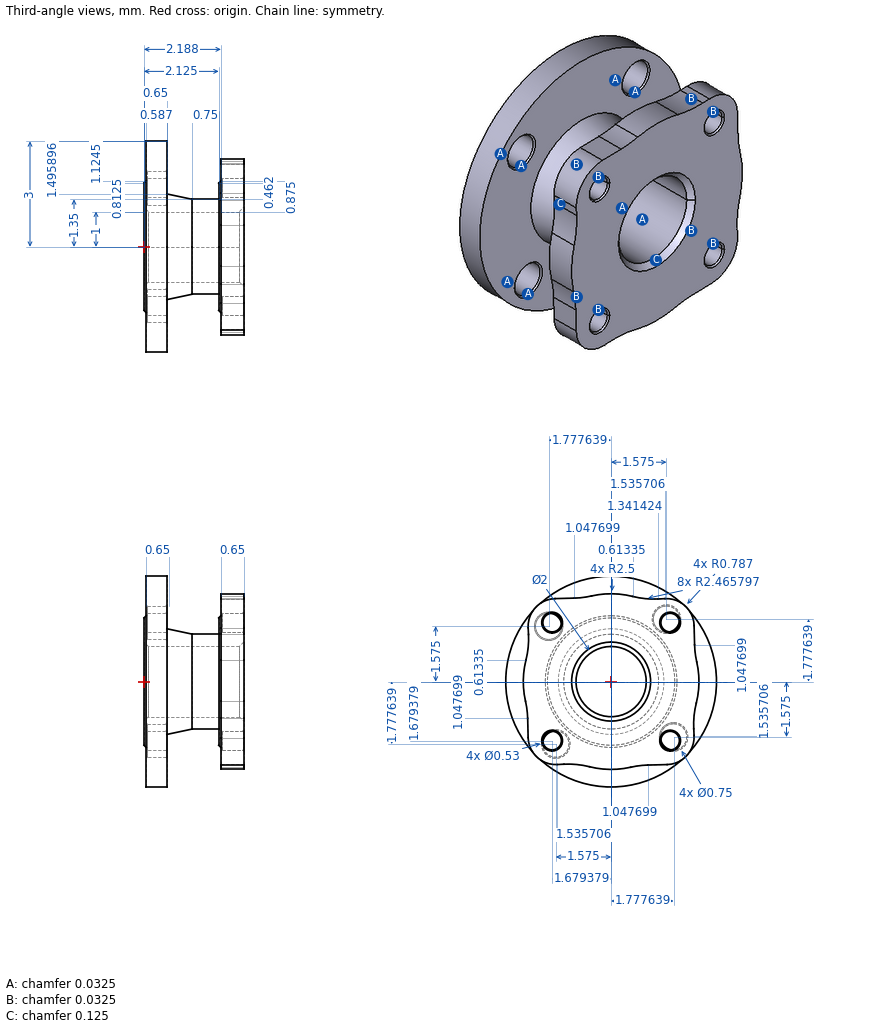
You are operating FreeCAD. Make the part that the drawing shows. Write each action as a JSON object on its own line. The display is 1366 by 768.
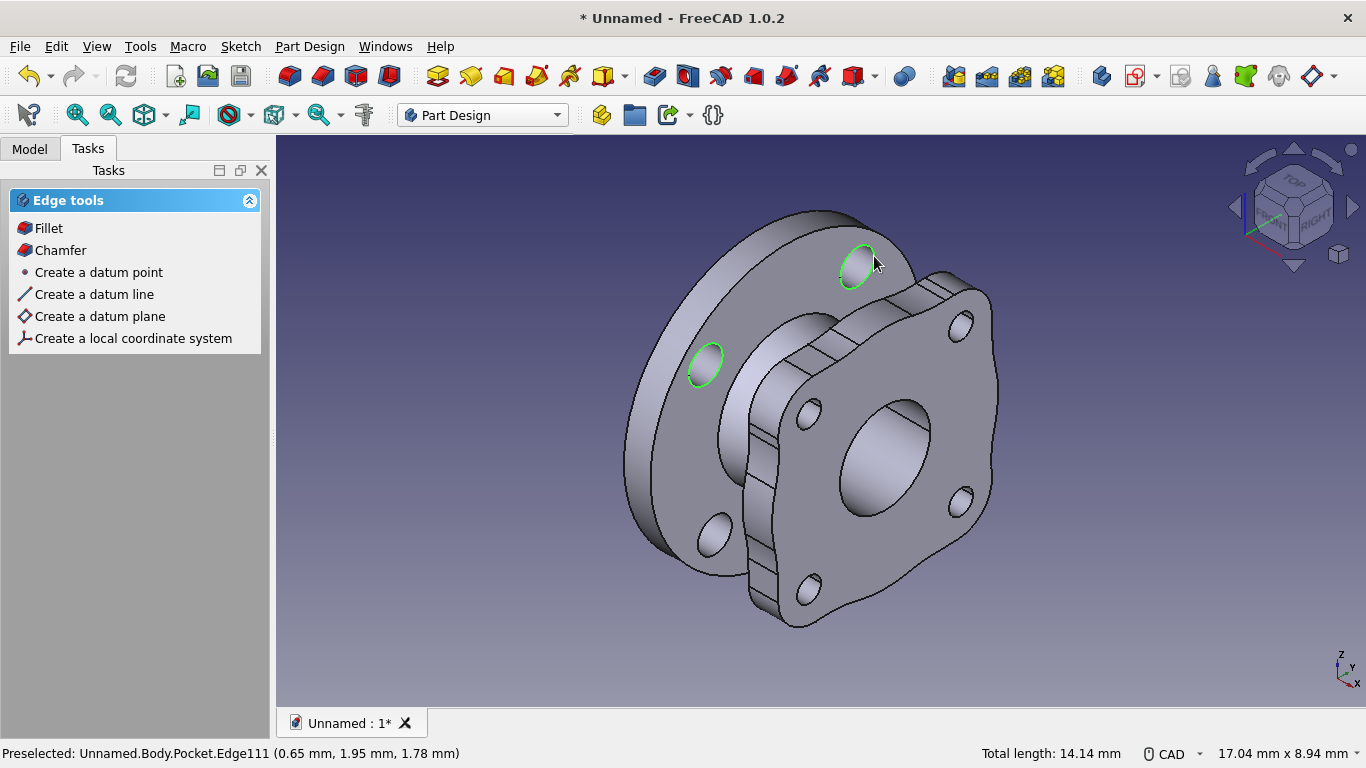
{"action": "left_click", "coordinate": [732, 524], "text": "ctrl"}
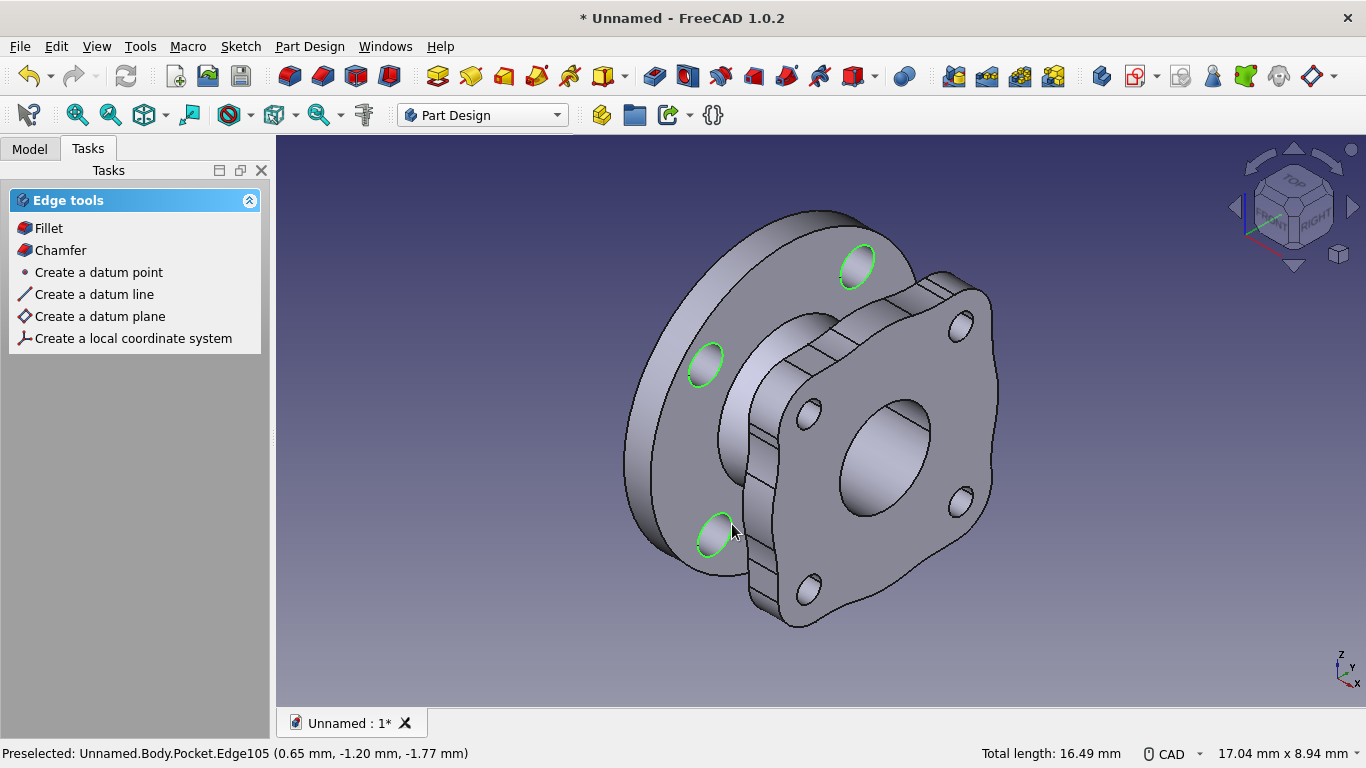
{"action": "key", "text": "2"}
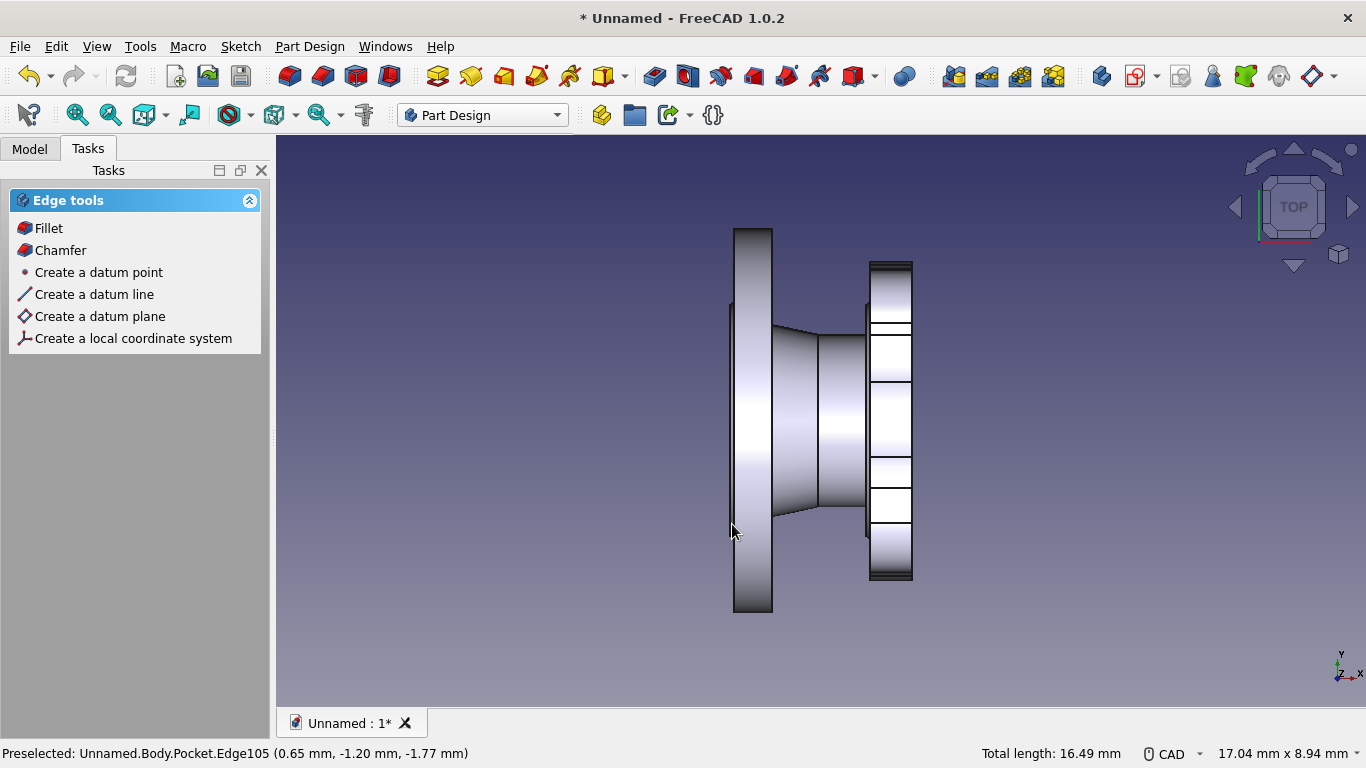
{"action": "key", "text": "1"}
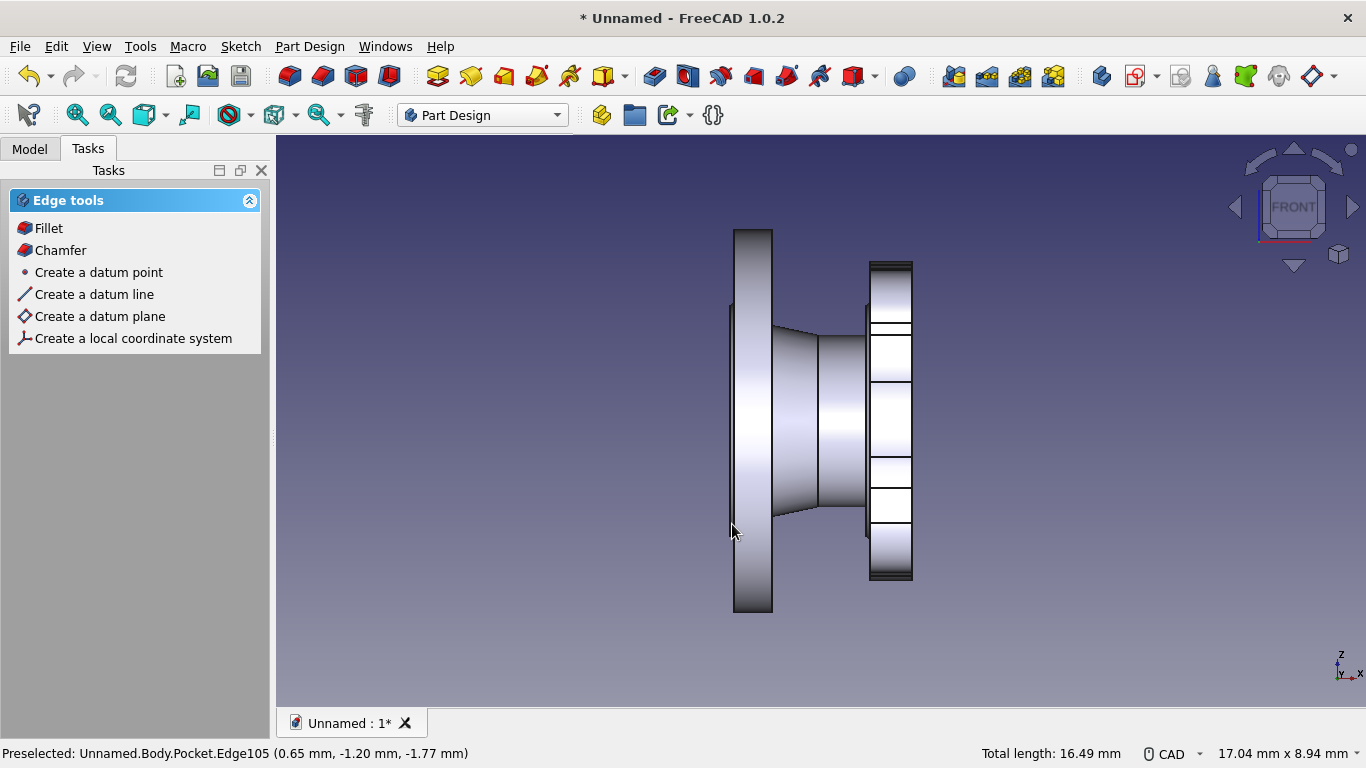
{"action": "key", "text": "3"}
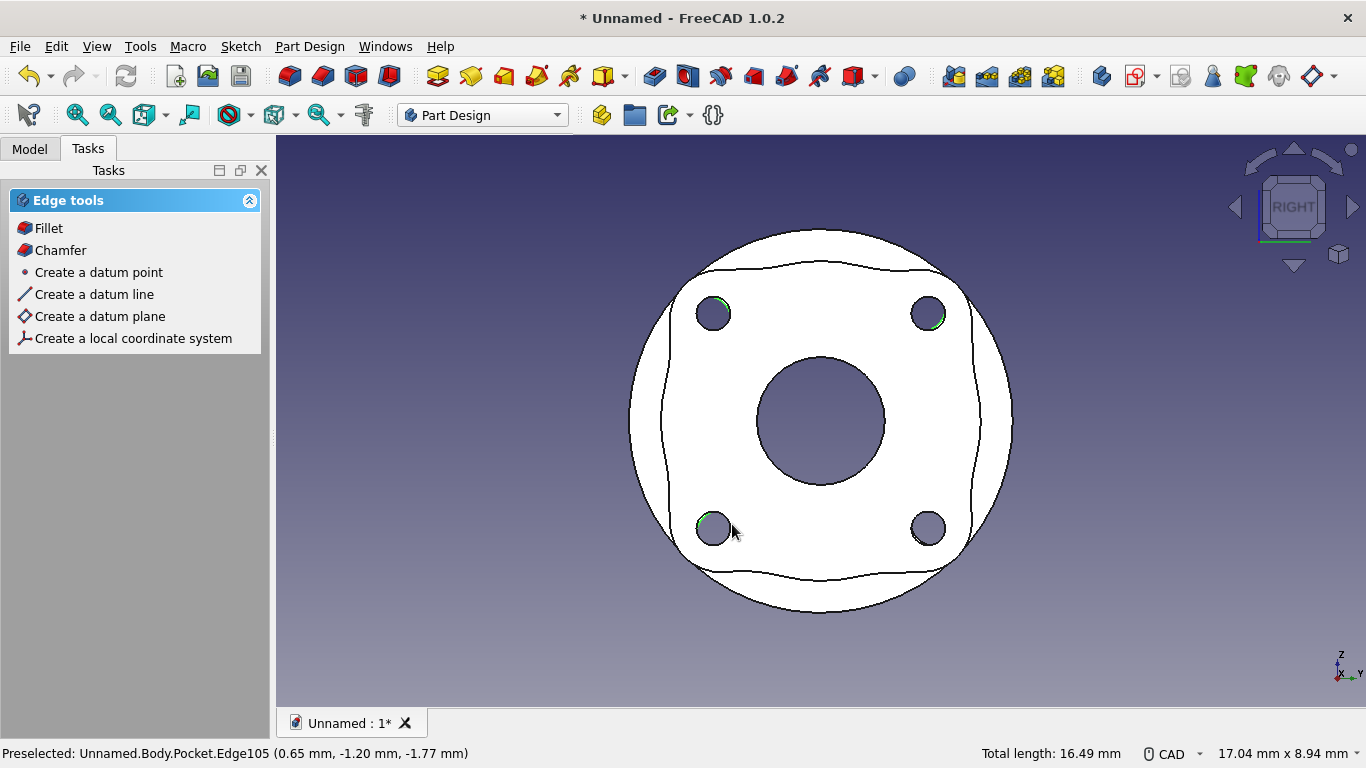
{"action": "key", "text": "5"}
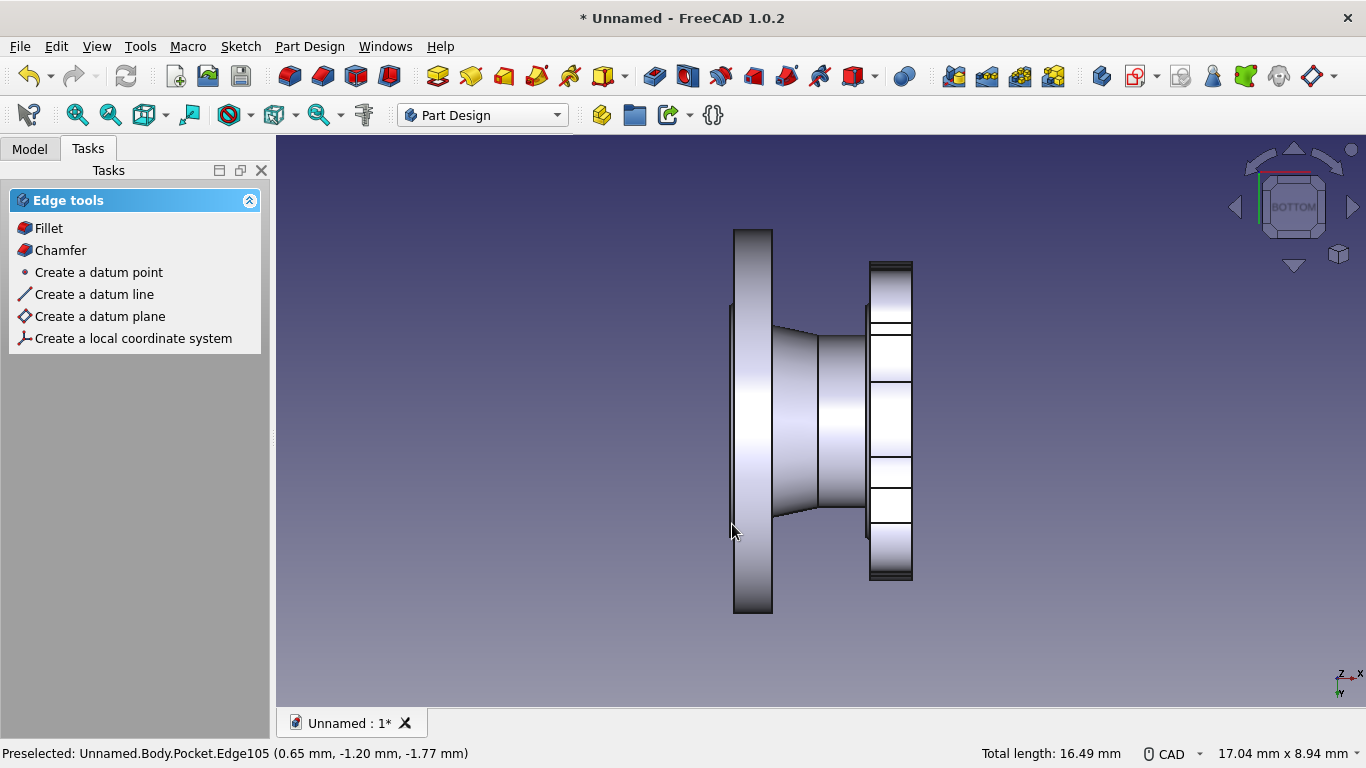
{"action": "key", "text": "4"}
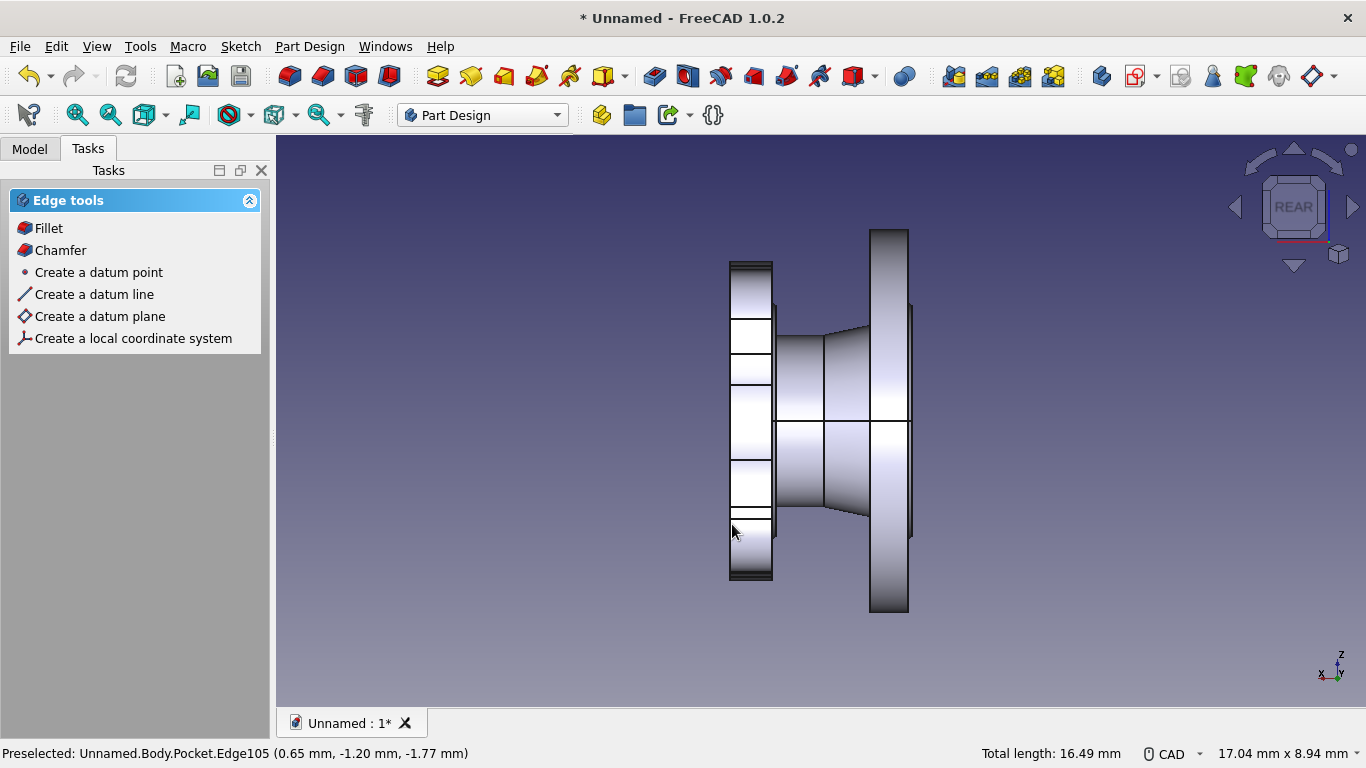
{"action": "key", "text": "6"}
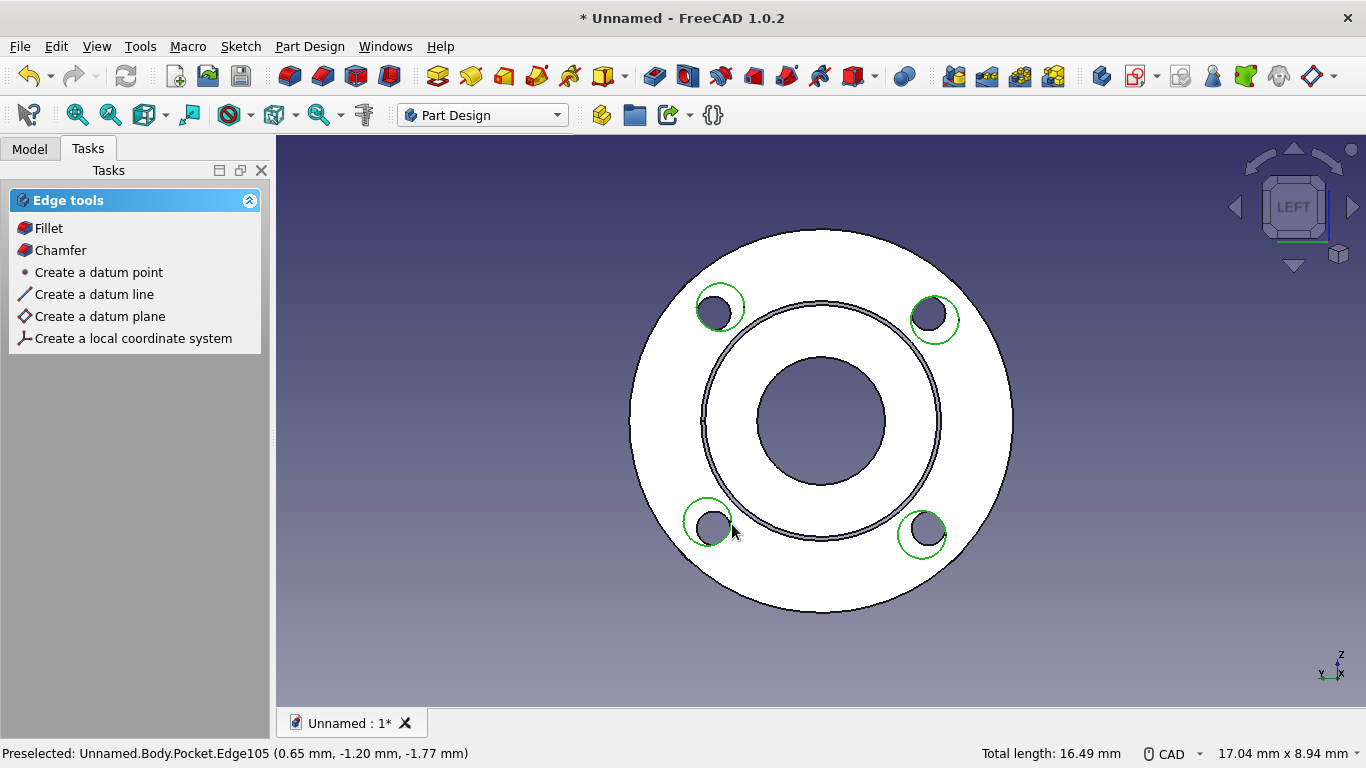
{"action": "key", "text": "v 3"}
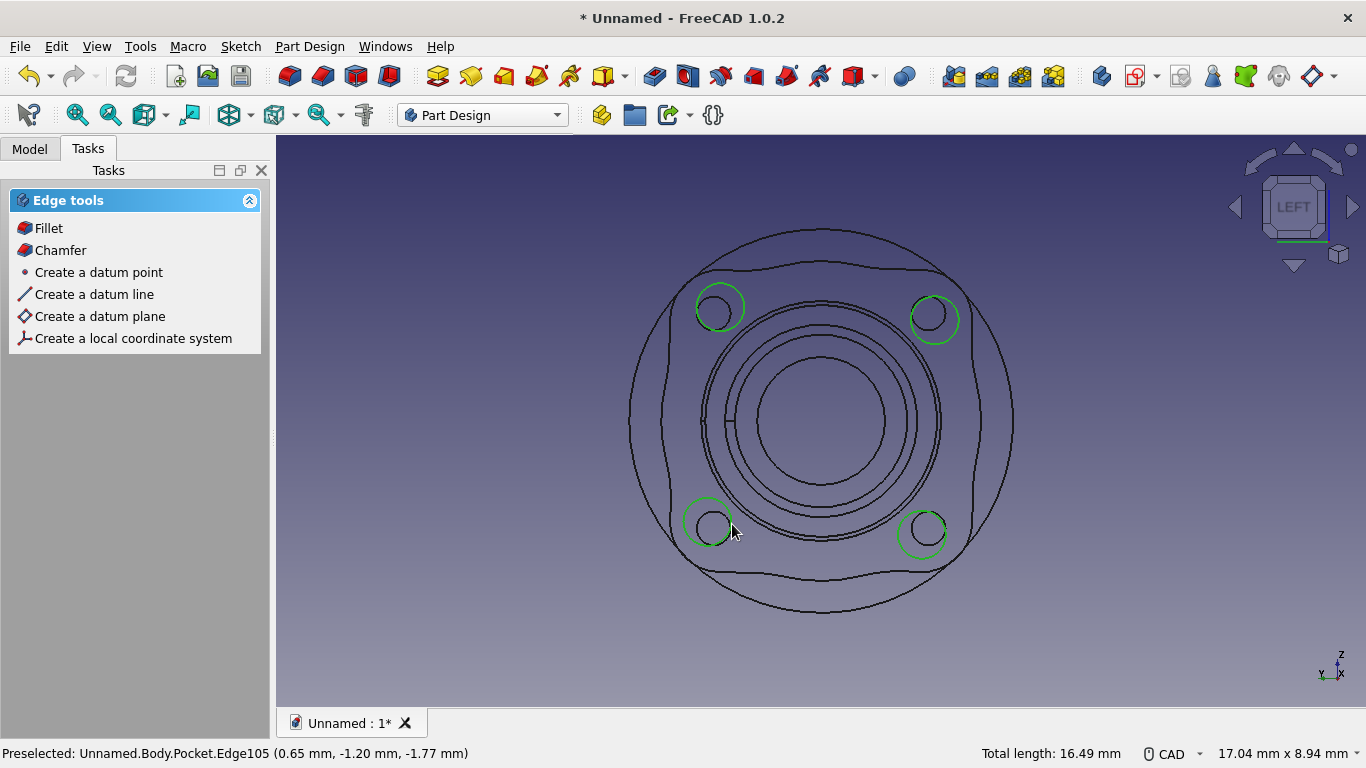
{"action": "key", "text": "0"}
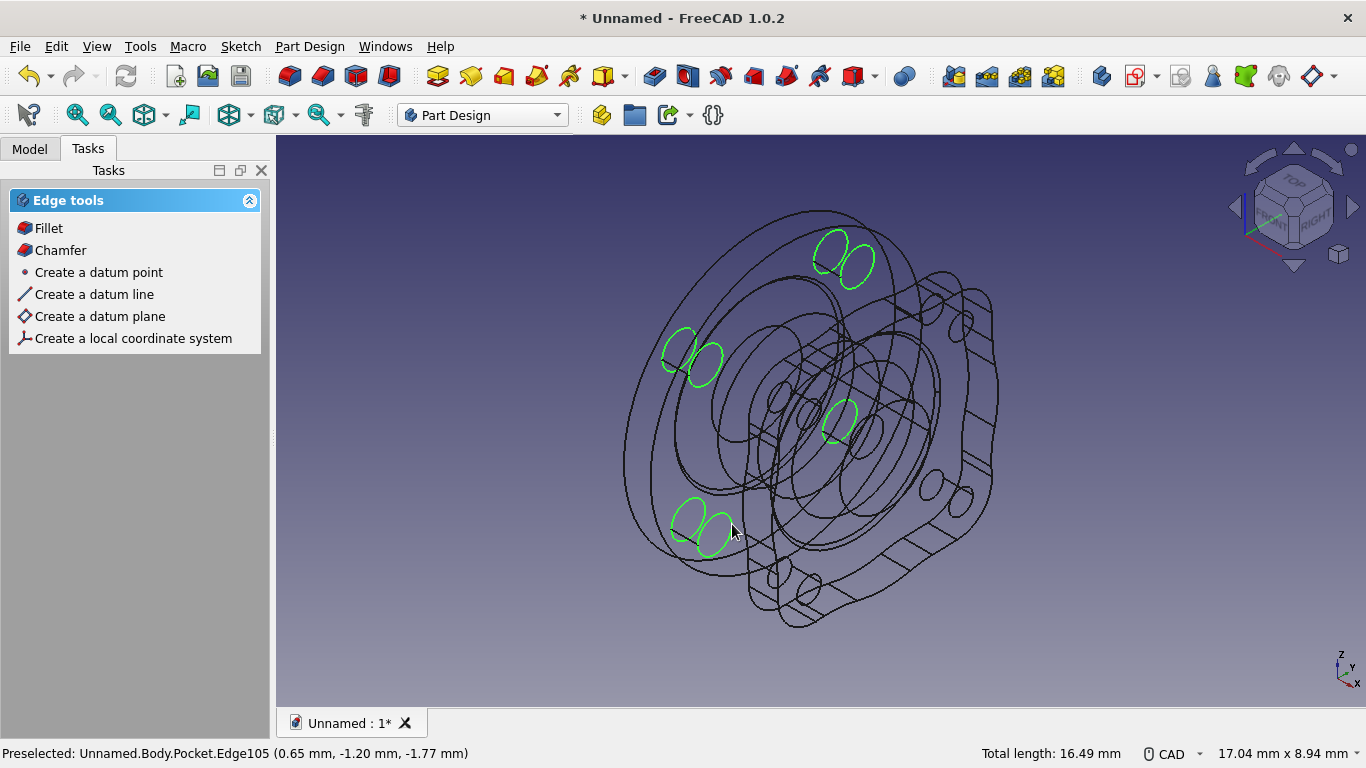
{"action": "left_click", "coordinate": [883, 426], "text": "ctrl"}